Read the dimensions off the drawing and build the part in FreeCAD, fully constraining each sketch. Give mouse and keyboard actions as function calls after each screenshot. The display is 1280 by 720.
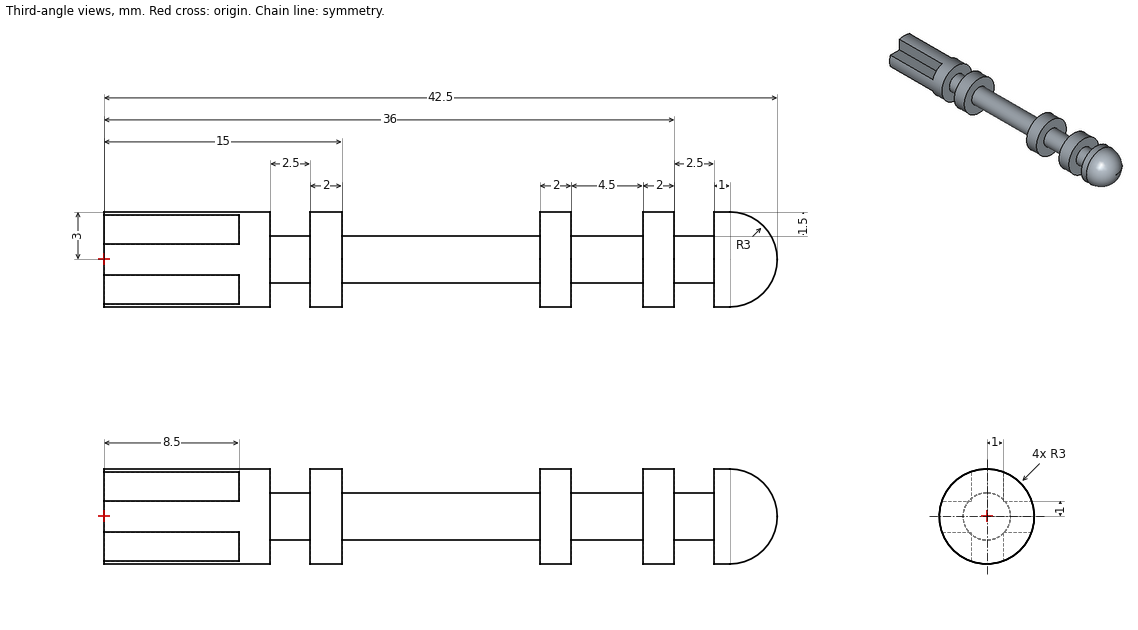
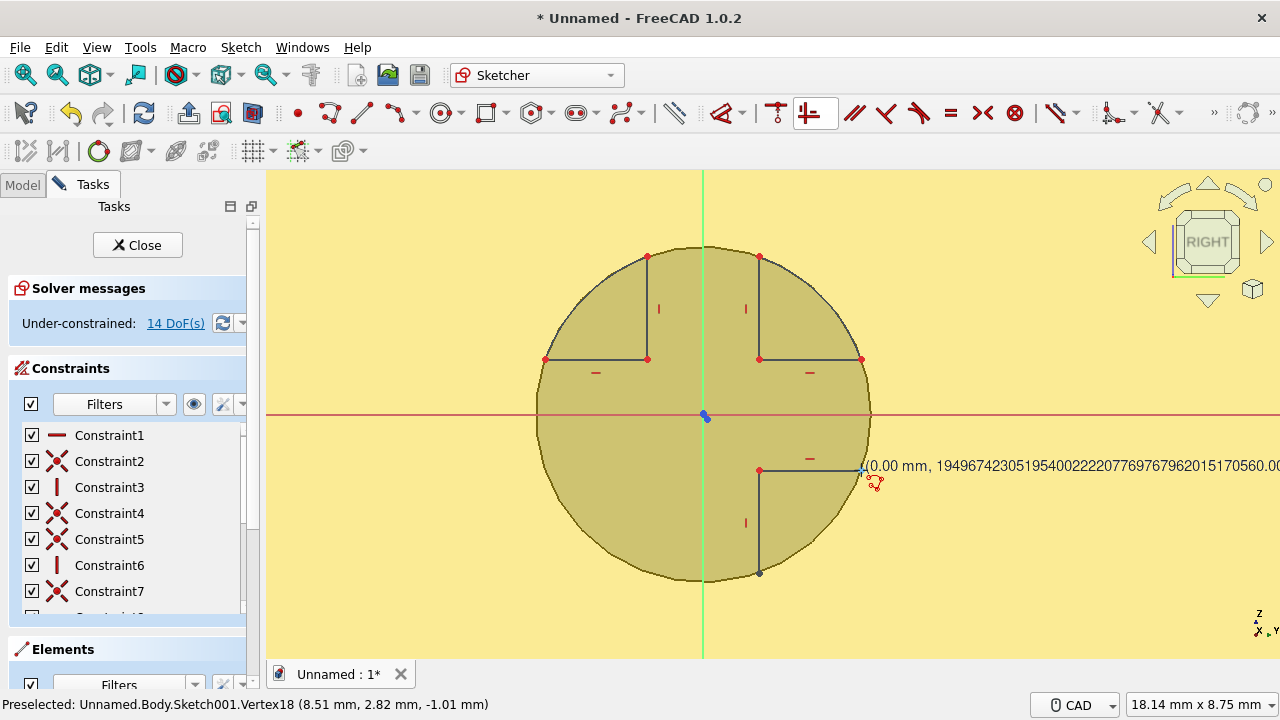
click(396, 114)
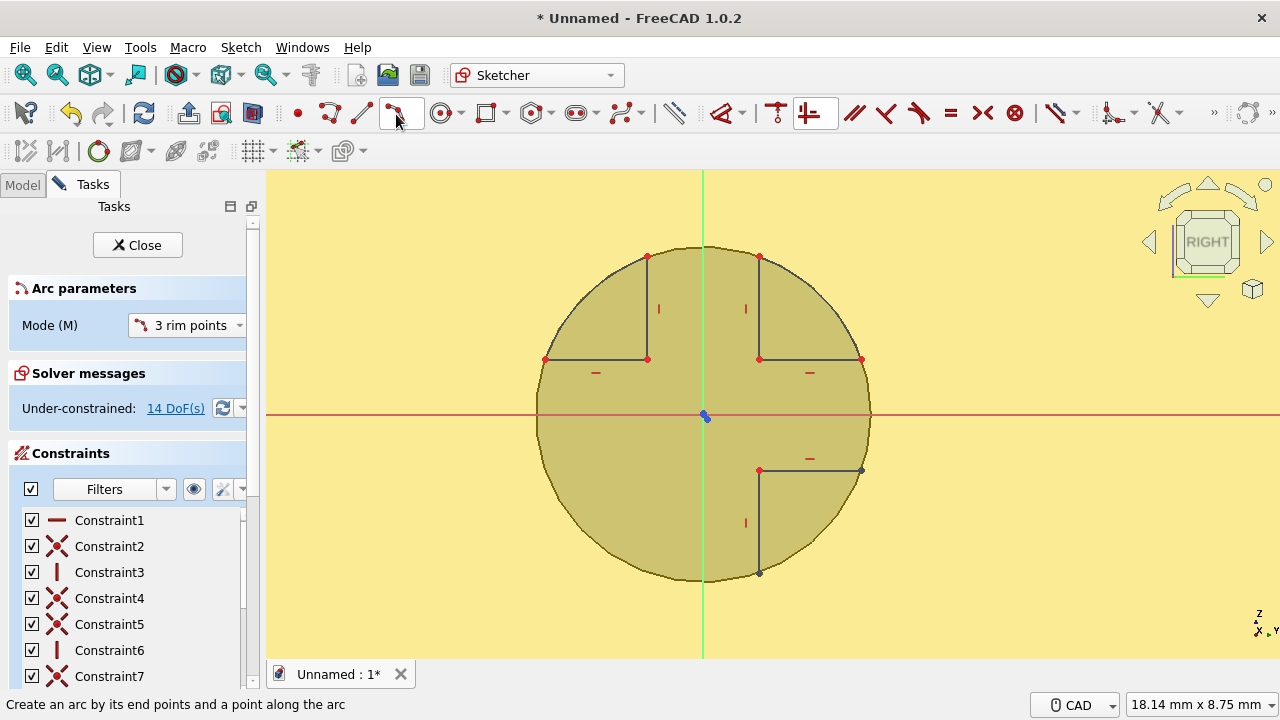
click(861, 471)
click(759, 574)
click(822, 533)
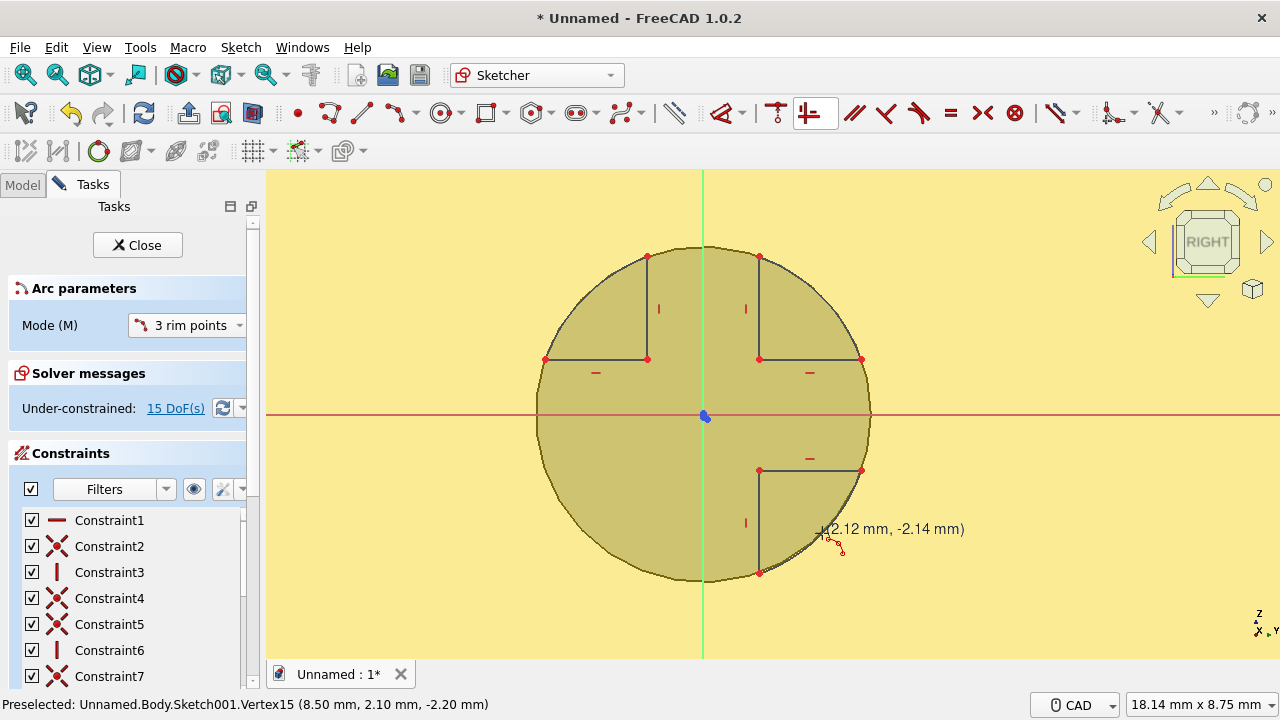
click(330, 114)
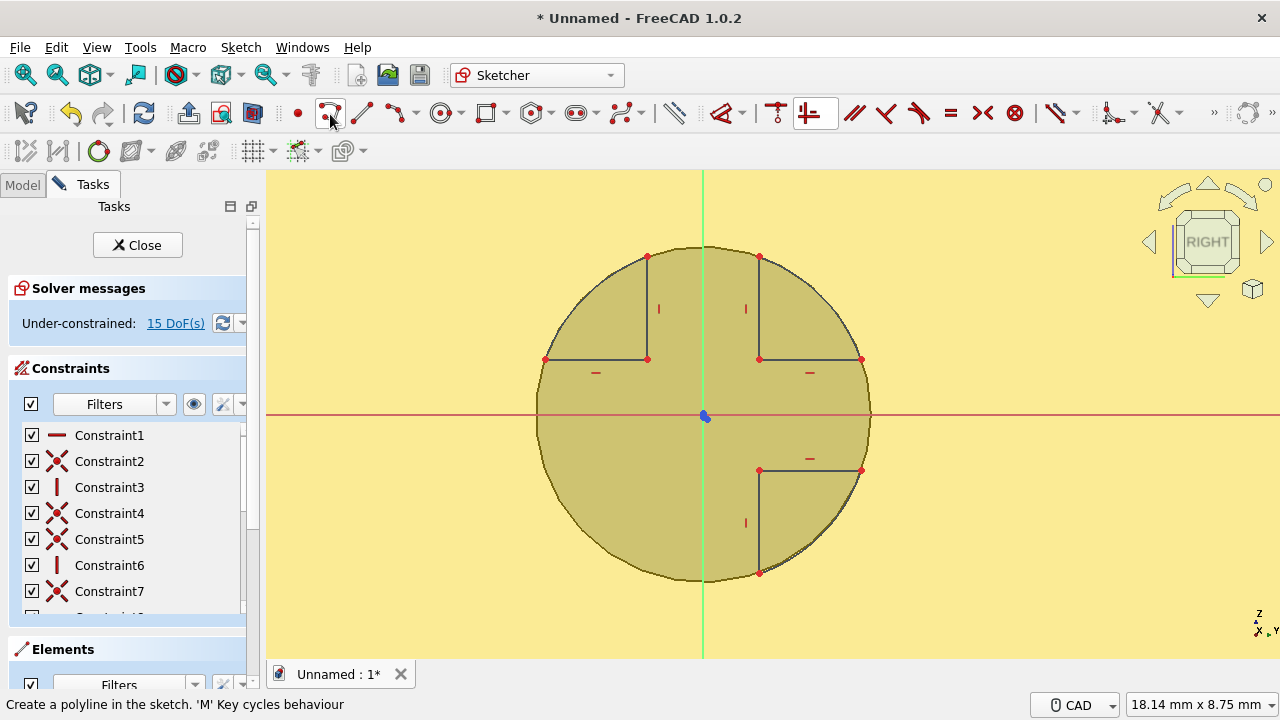
click(545, 470)
click(647, 470)
click(647, 573)
right_click(647, 573)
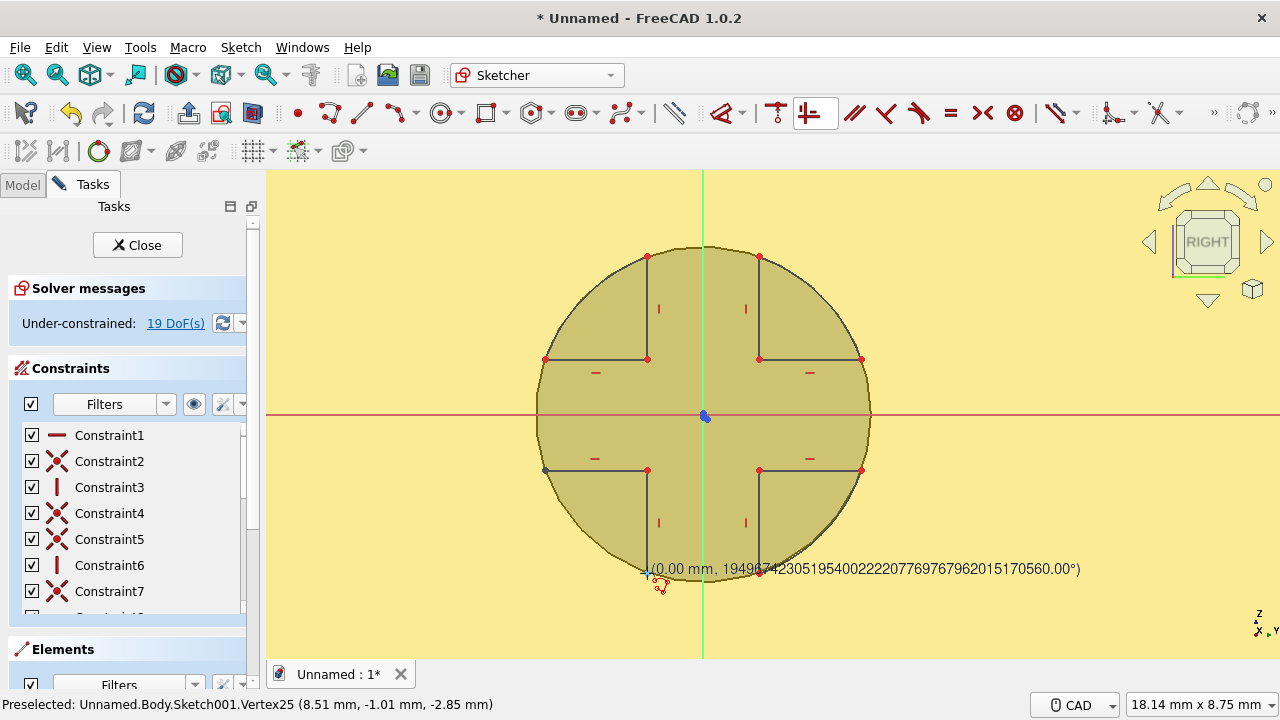
click(396, 114)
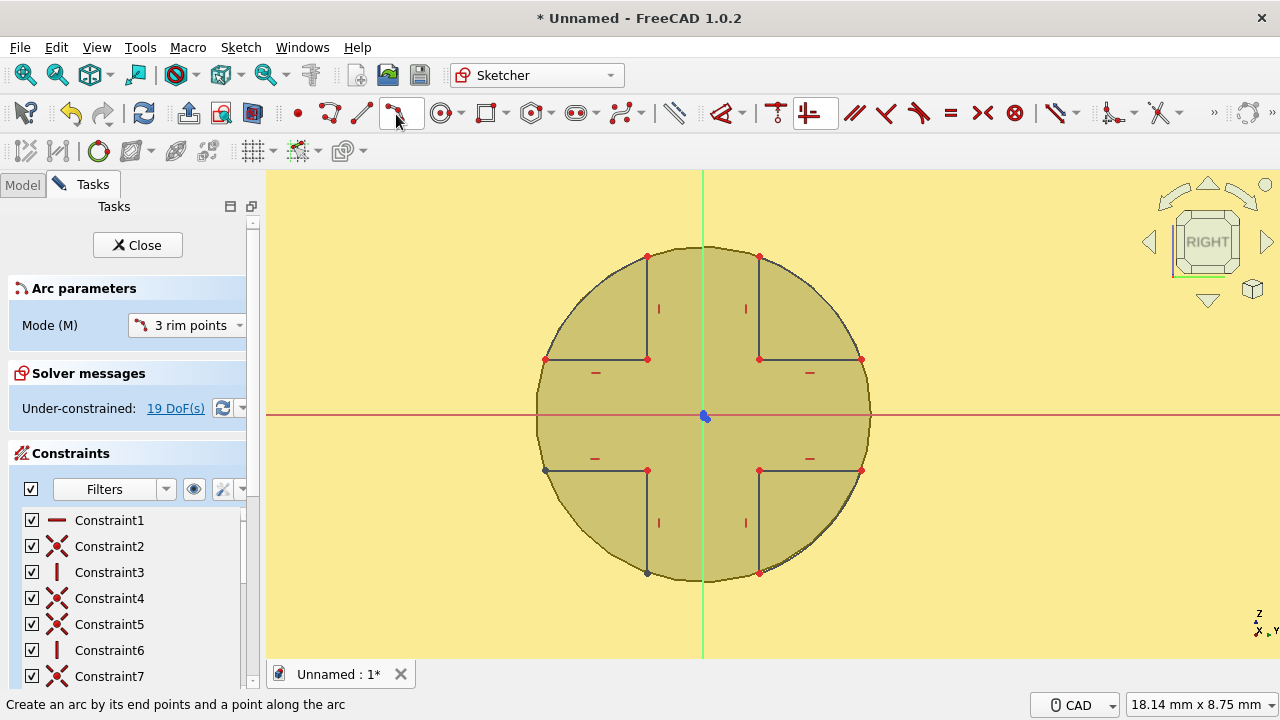
click(647, 574)
click(545, 471)
click(585, 533)
key(Escape)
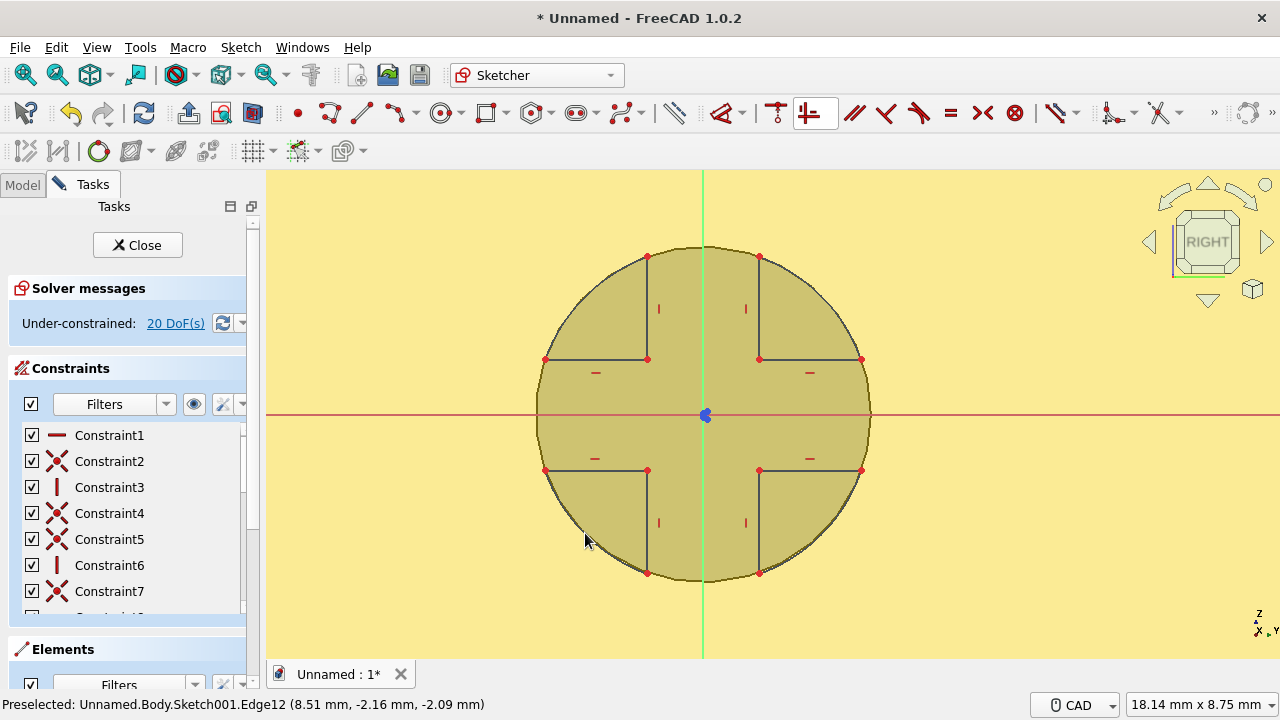
click(841, 320)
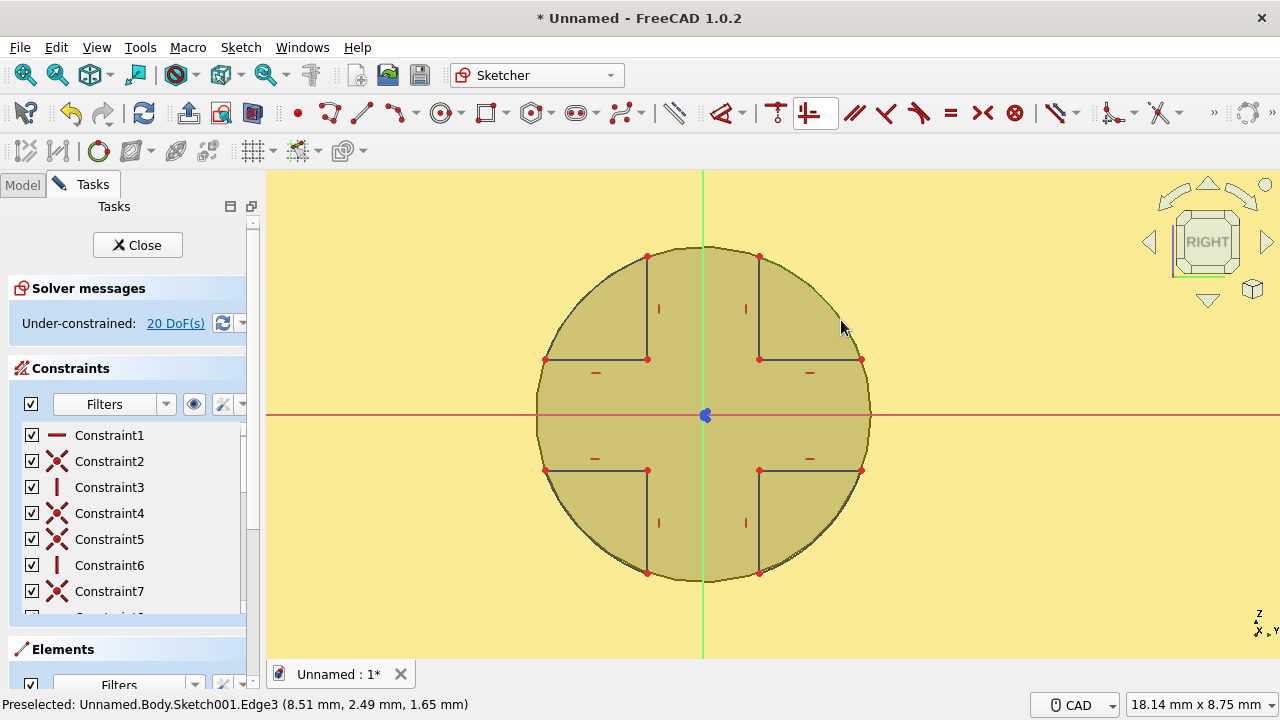
click(607, 278)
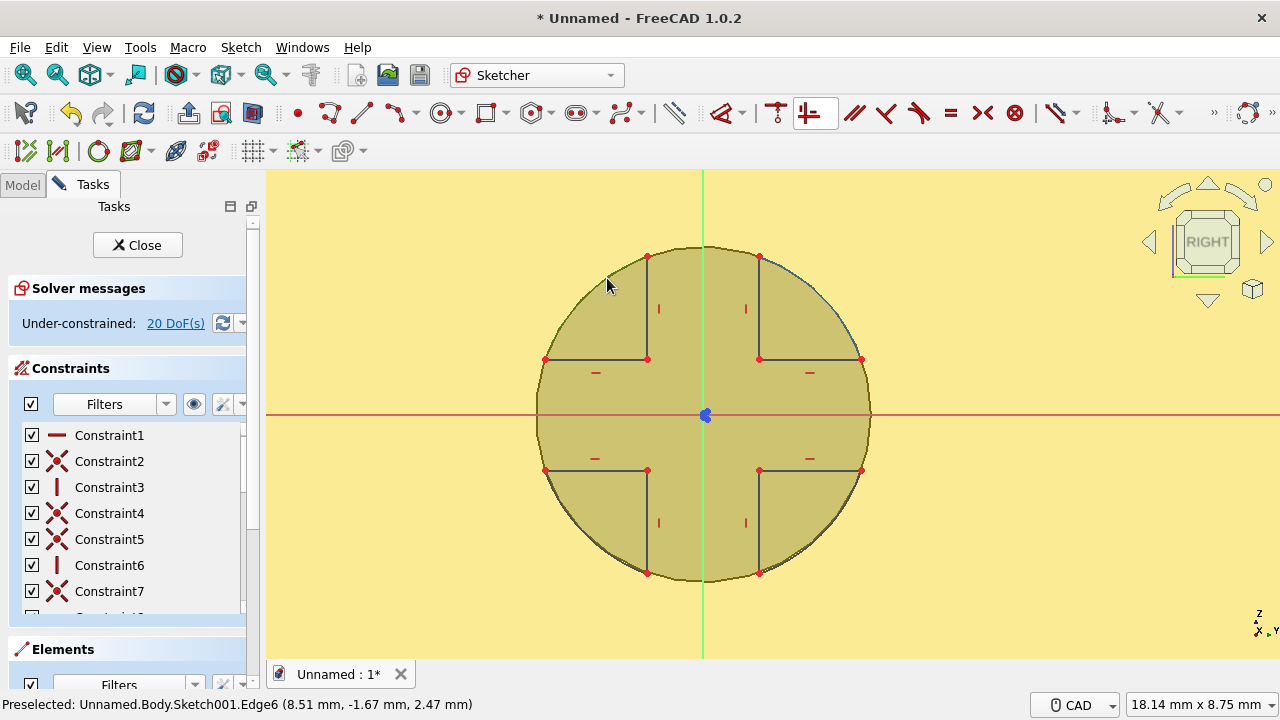
click(776, 114)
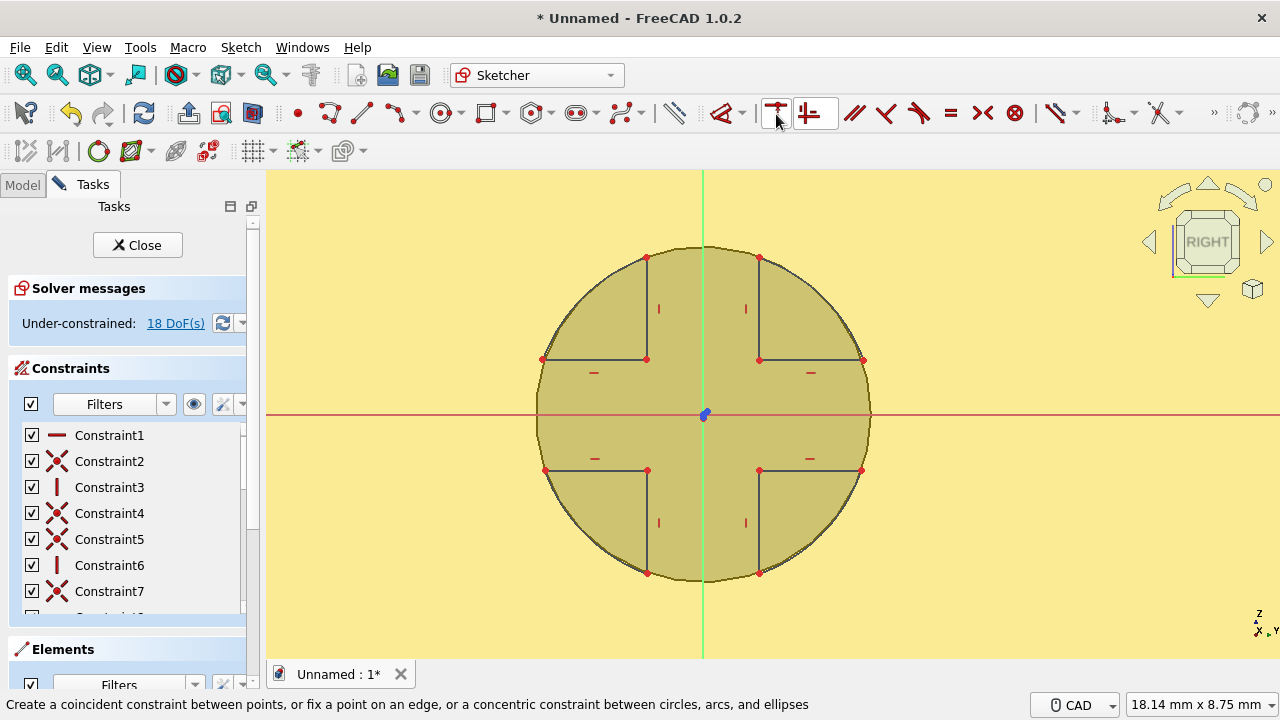
click(842, 320)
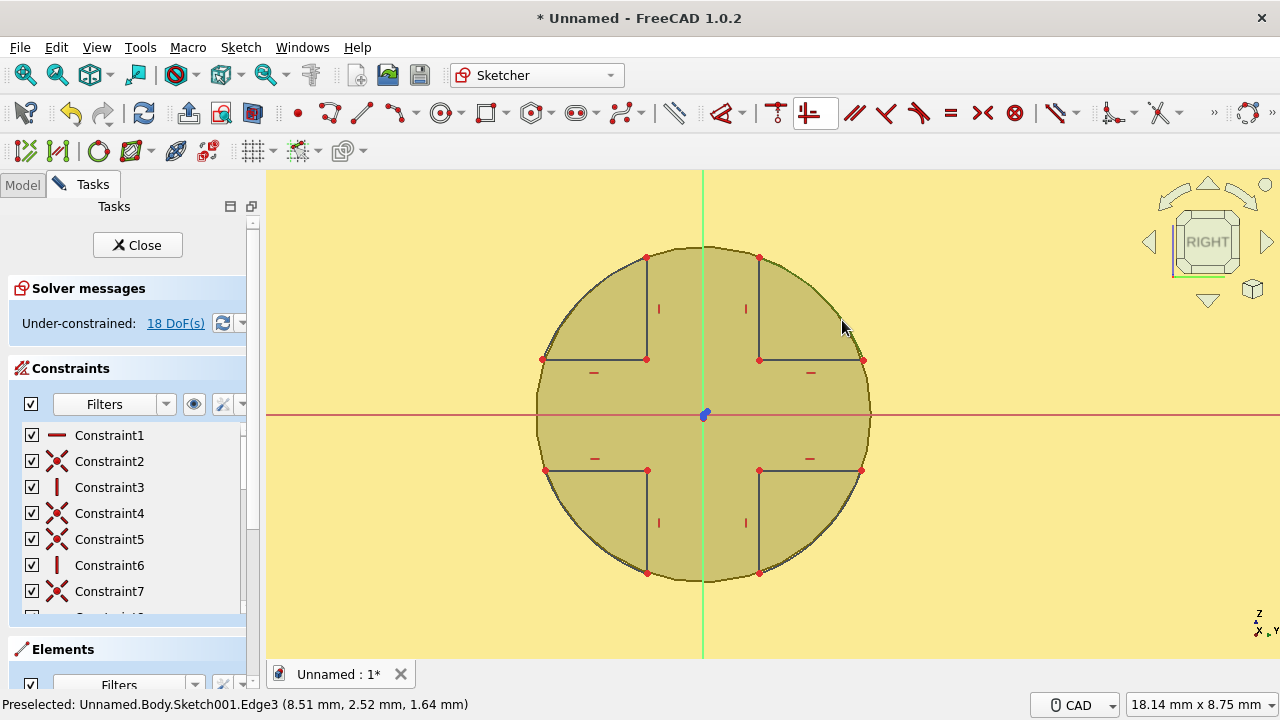
click(799, 553)